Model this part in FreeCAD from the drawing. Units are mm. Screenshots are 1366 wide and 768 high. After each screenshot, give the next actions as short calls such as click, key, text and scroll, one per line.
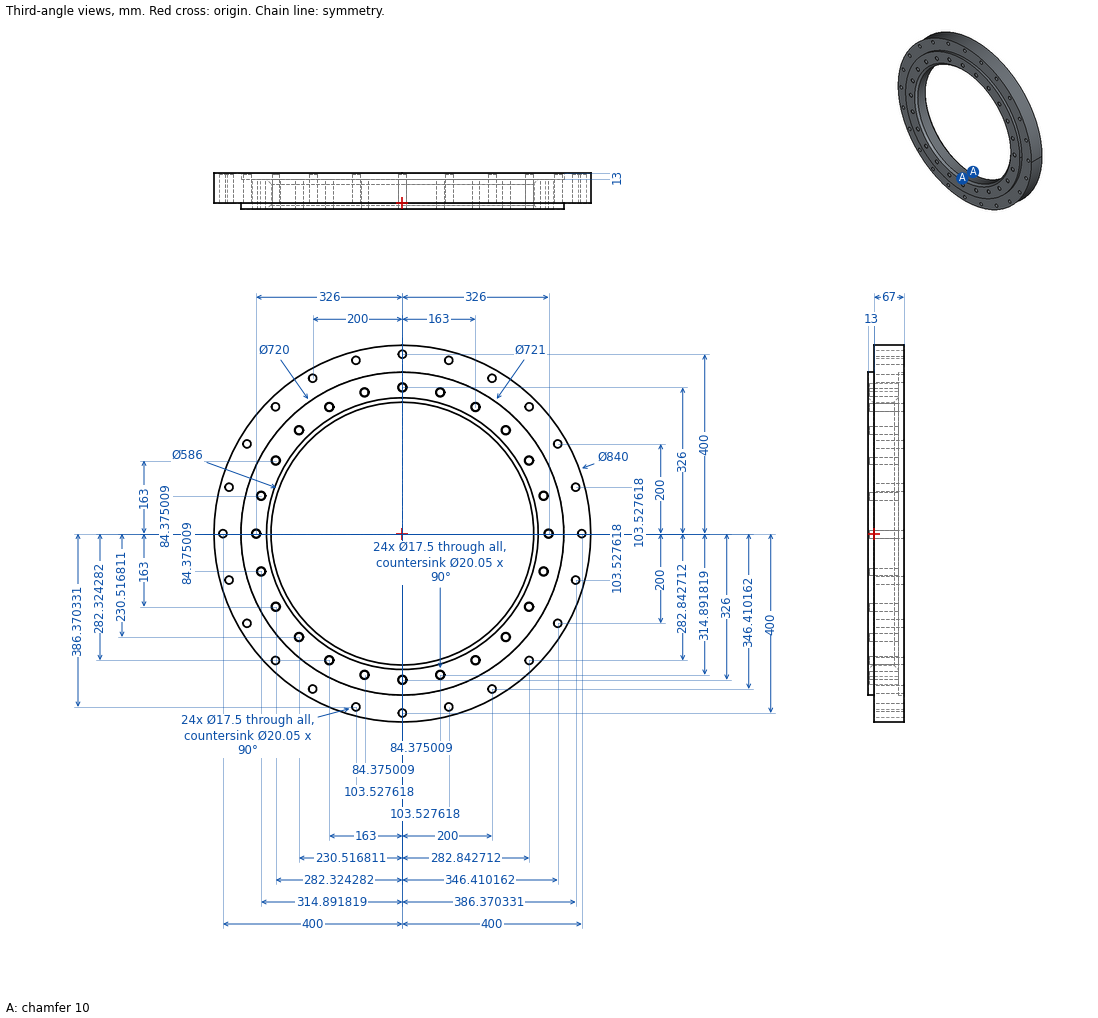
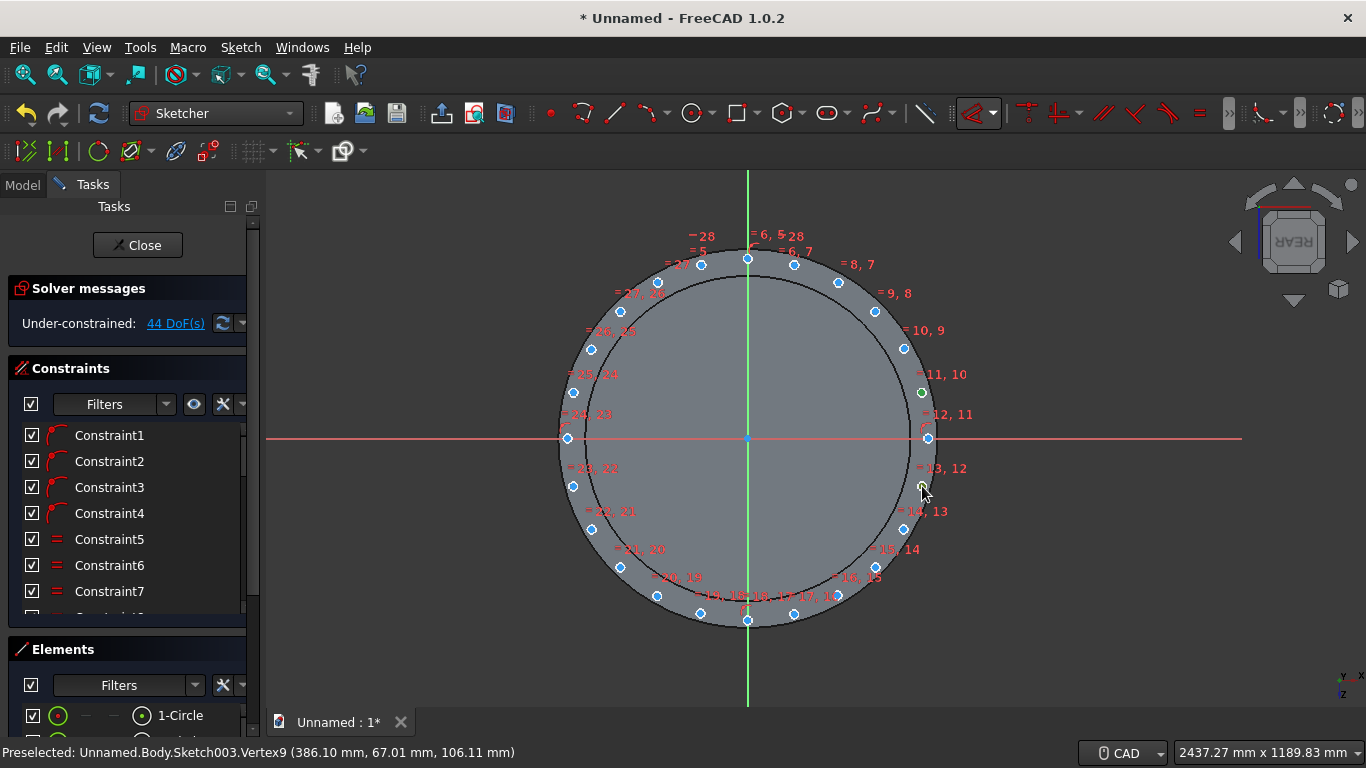
key(v)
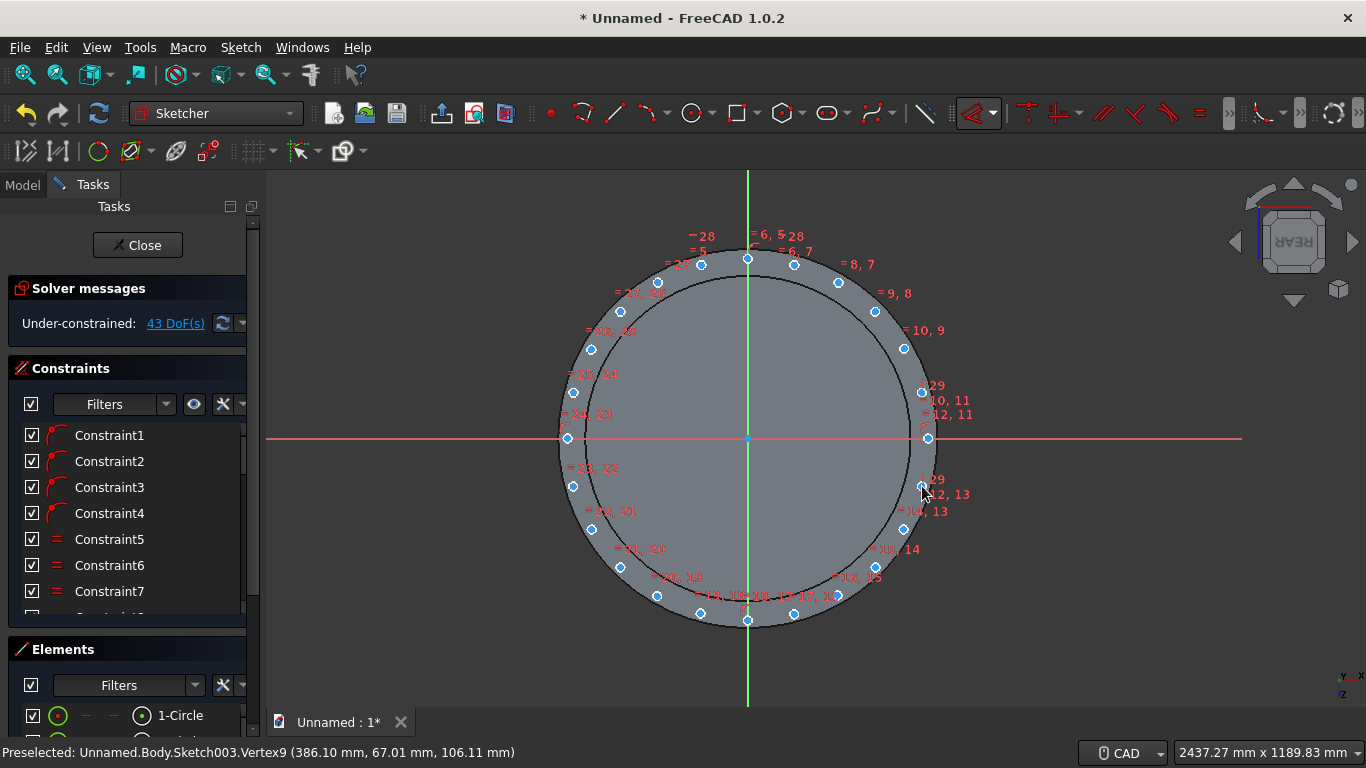
click(904, 349)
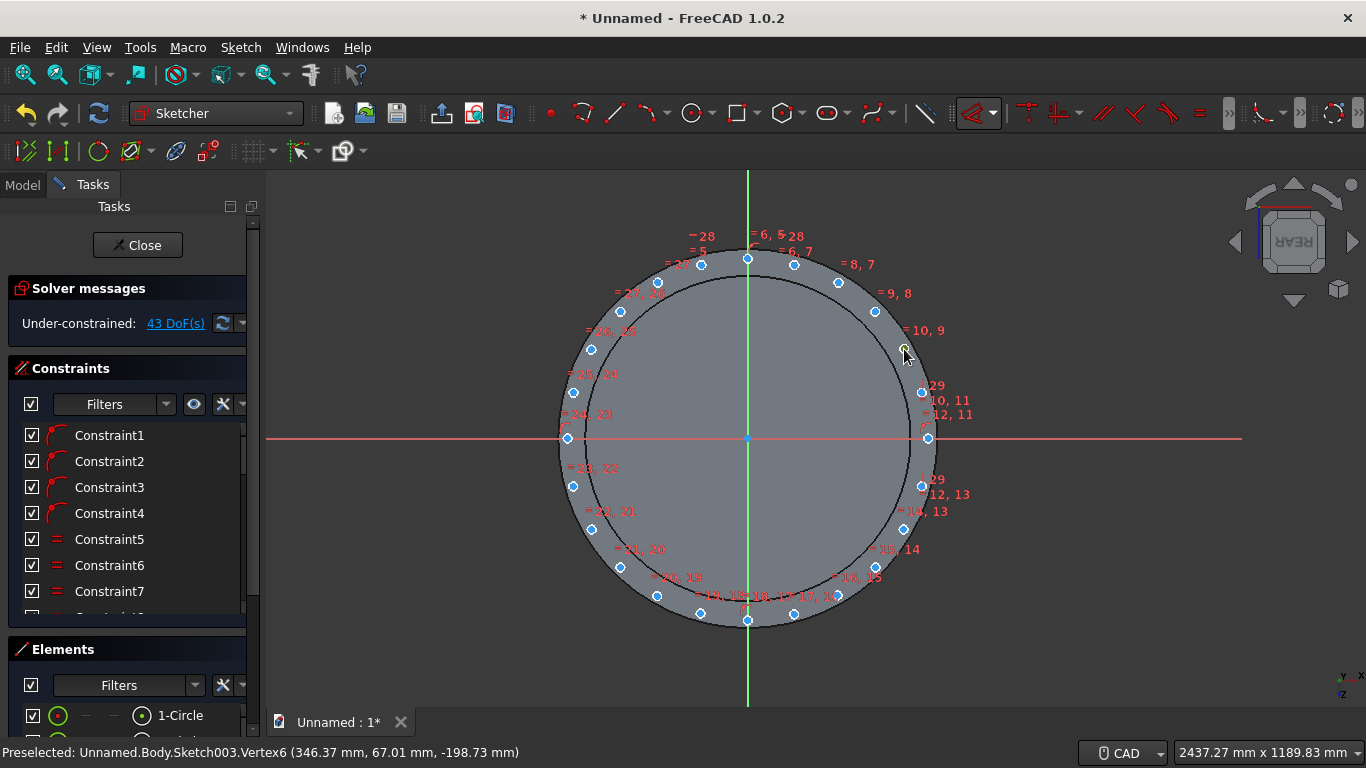
click(904, 530)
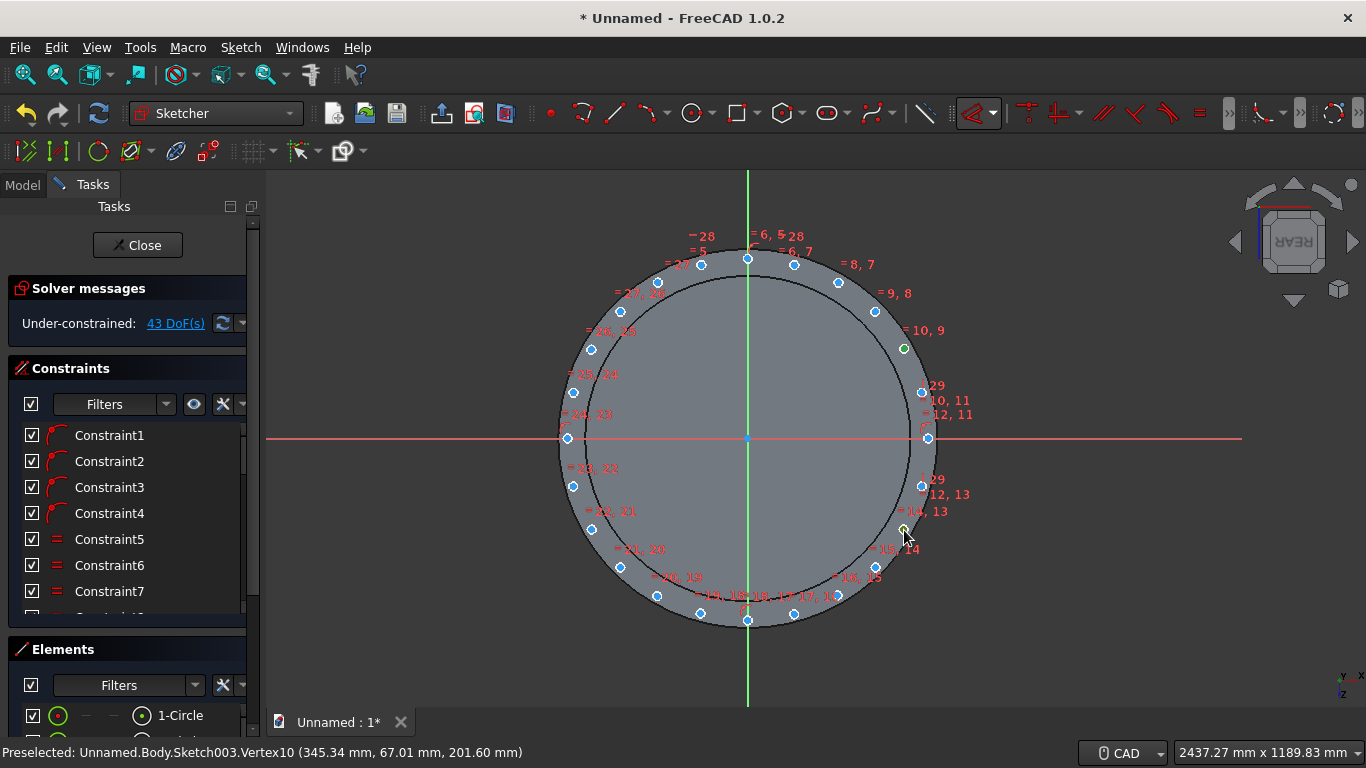
key(v)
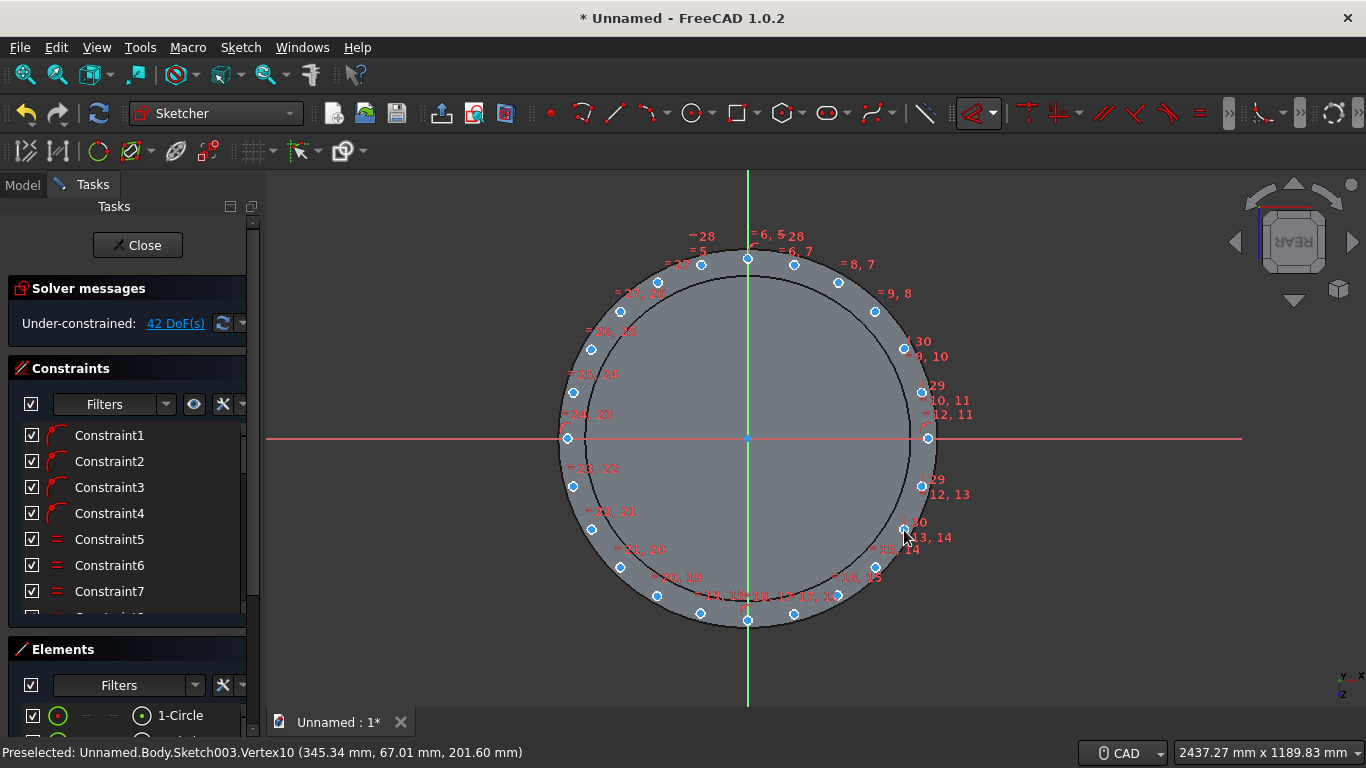
click(875, 312)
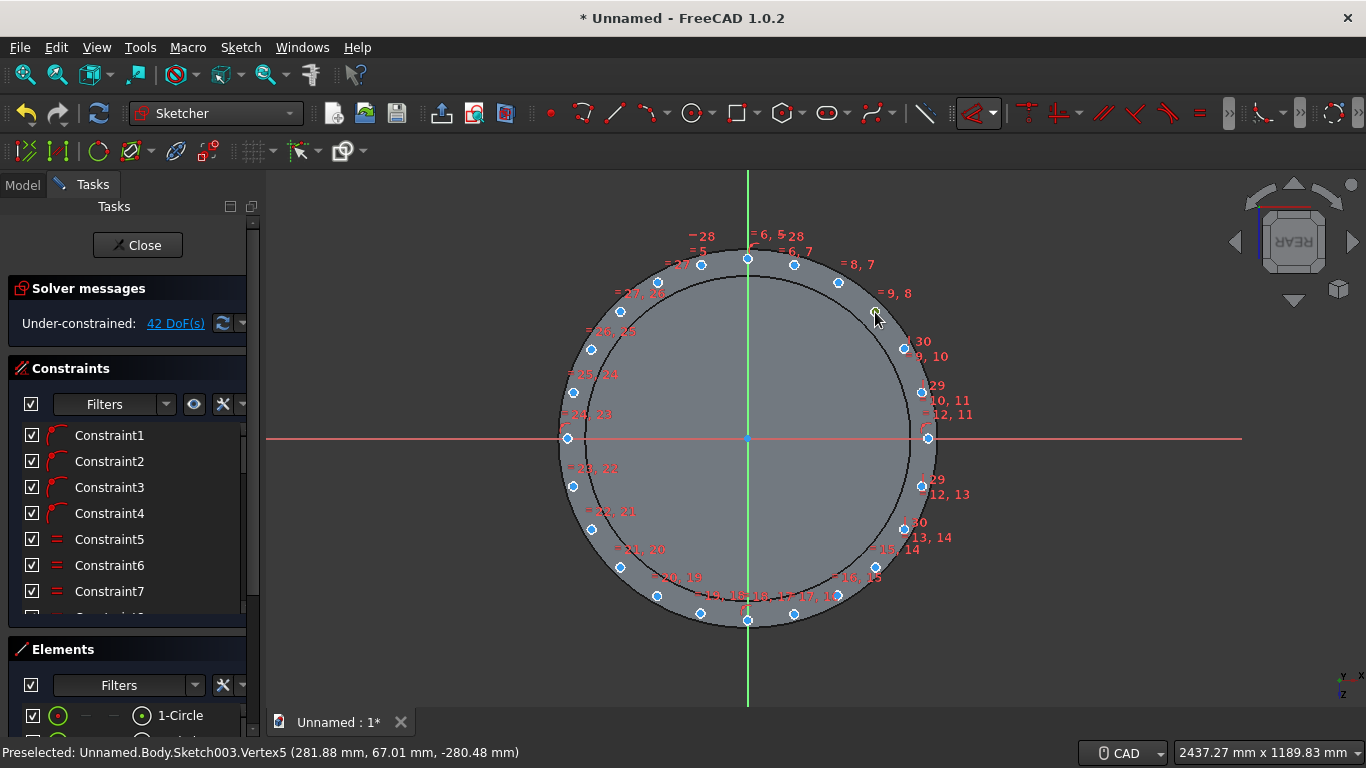
click(876, 568)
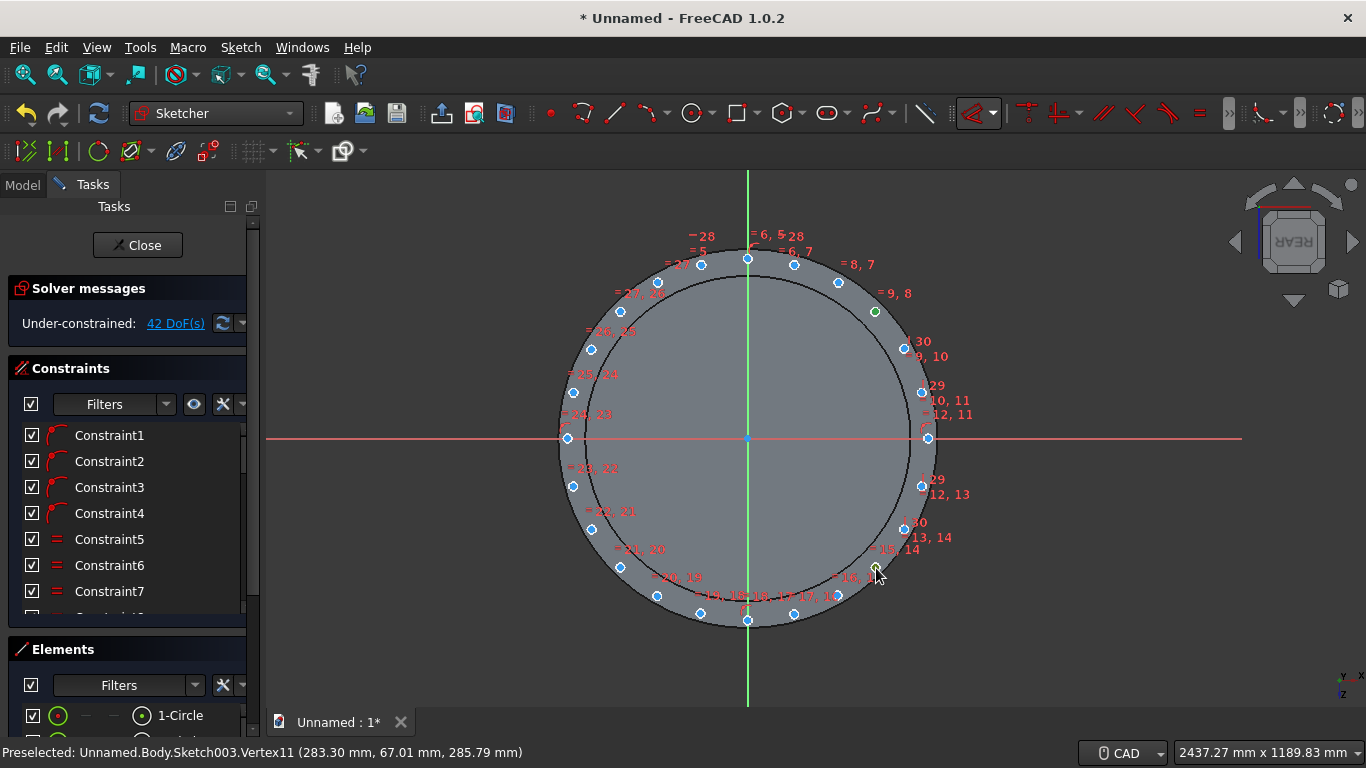
key(v)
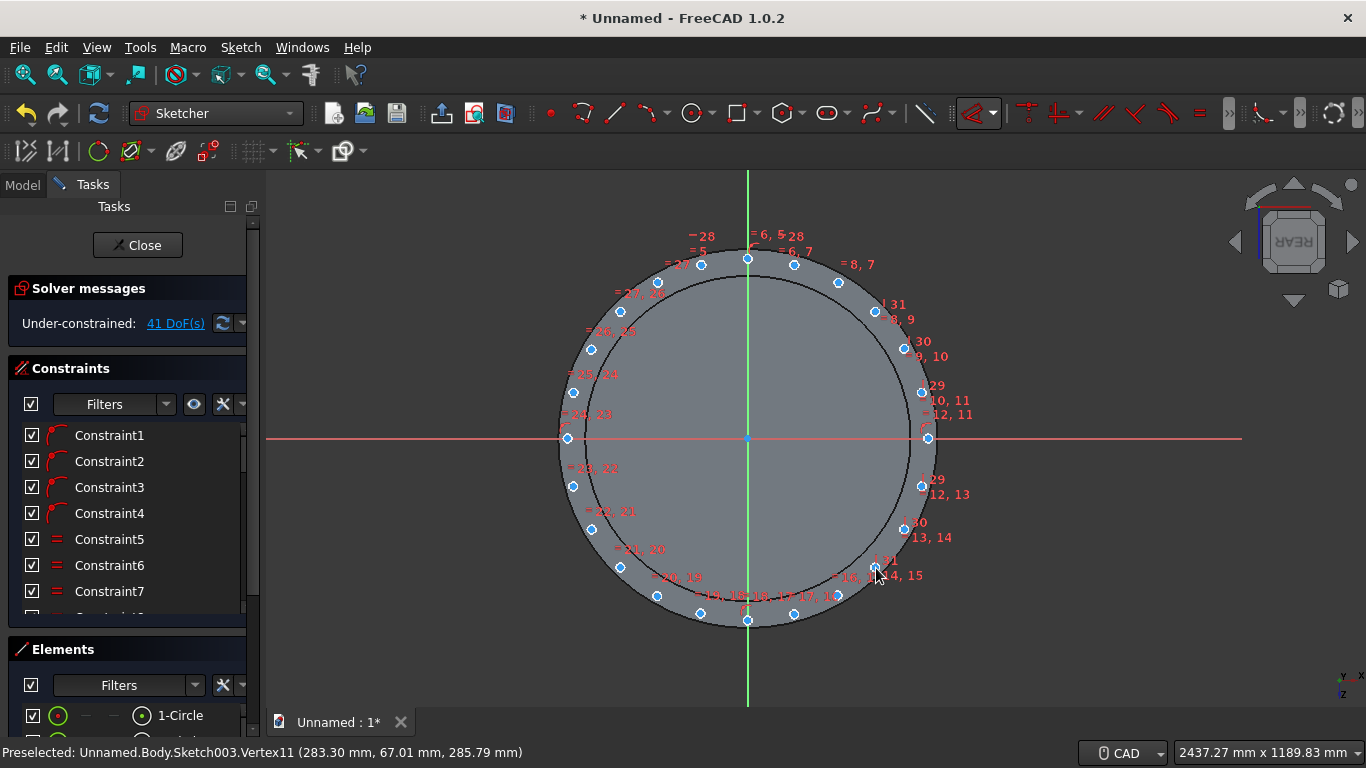
click(794, 614)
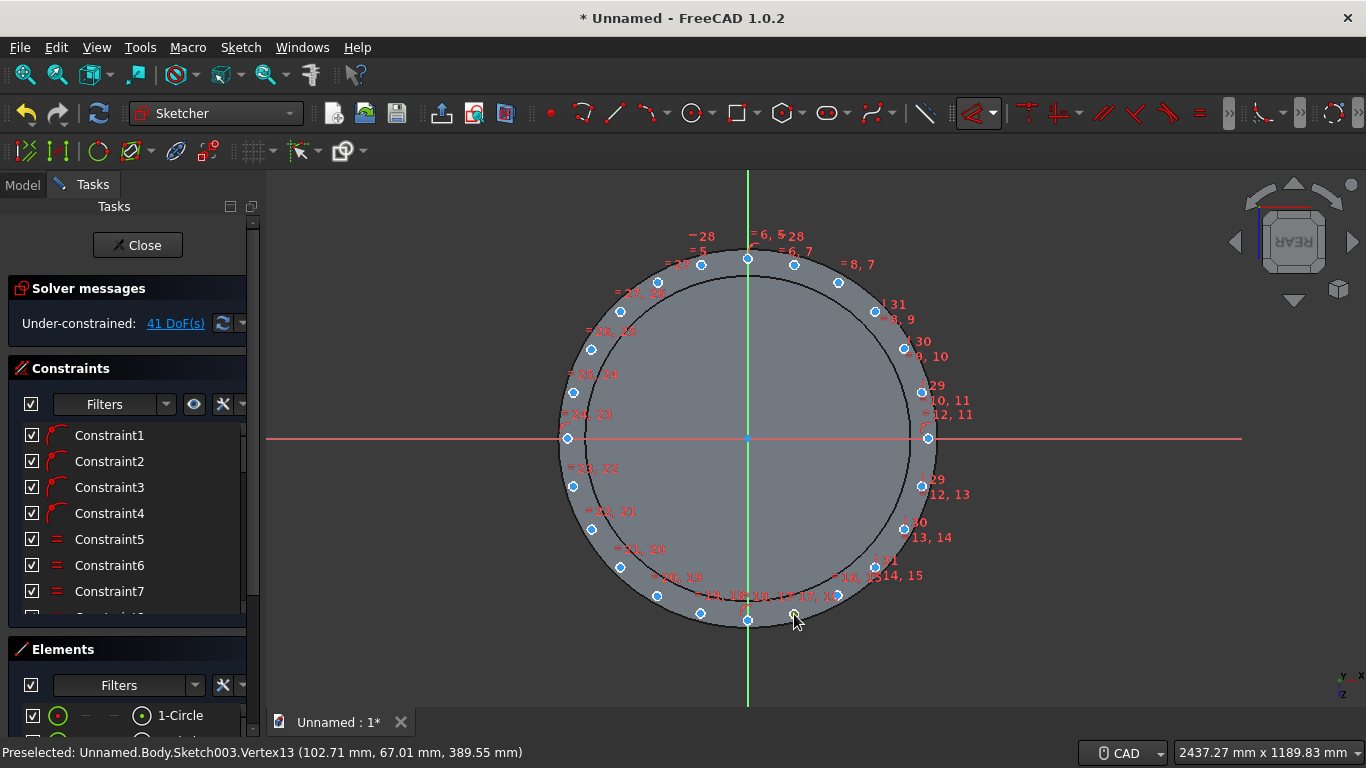
click(701, 614)